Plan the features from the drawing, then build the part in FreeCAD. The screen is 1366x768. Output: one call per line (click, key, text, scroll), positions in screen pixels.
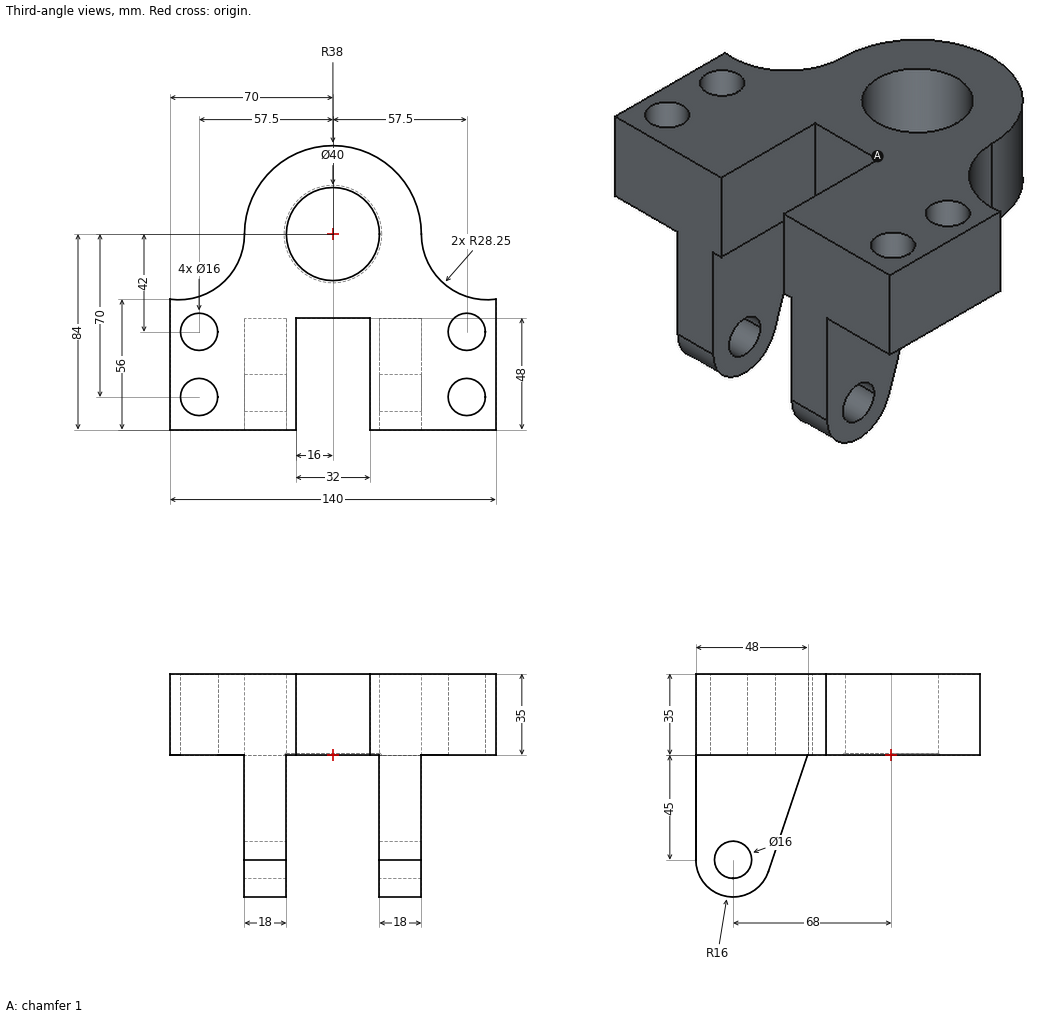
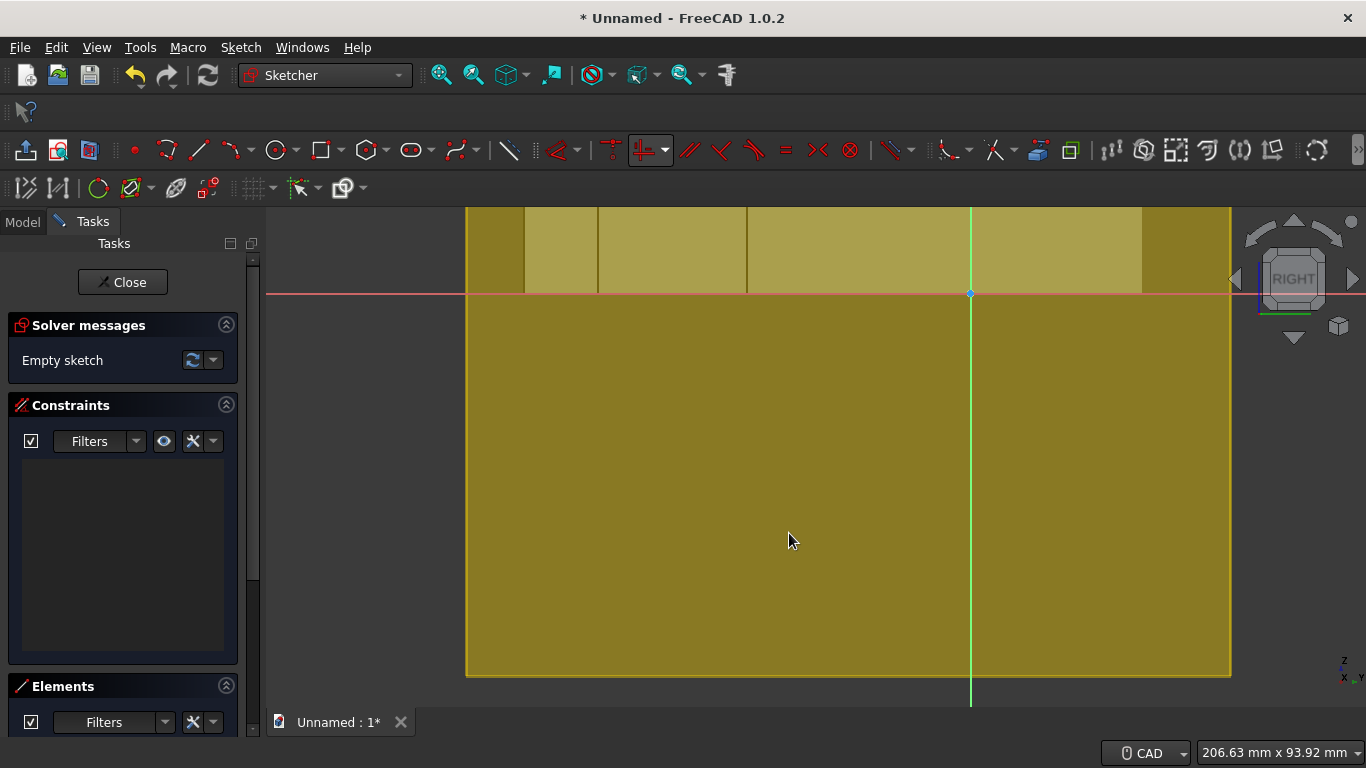
click(168, 150)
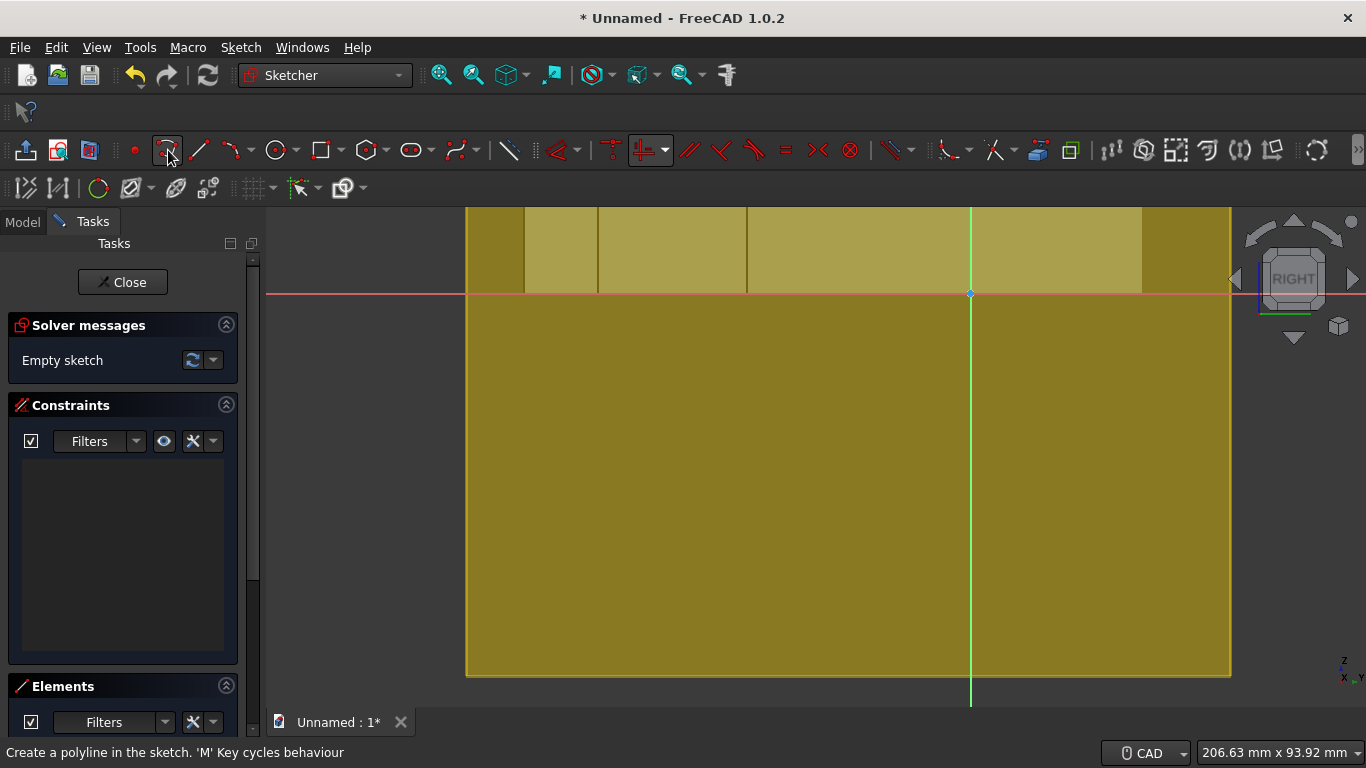
click(690, 561)
click(779, 294)
click(524, 303)
click(524, 534)
right_click(524, 534)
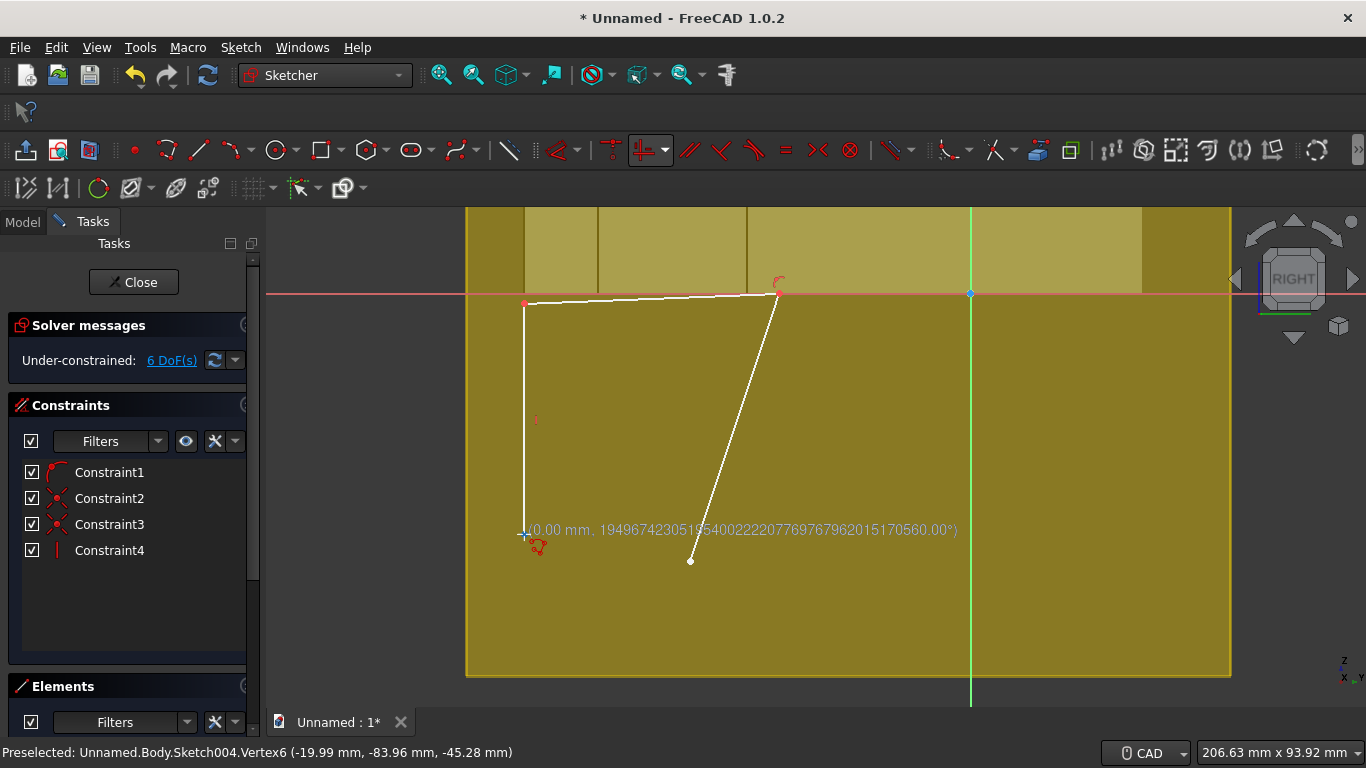
click(232, 150)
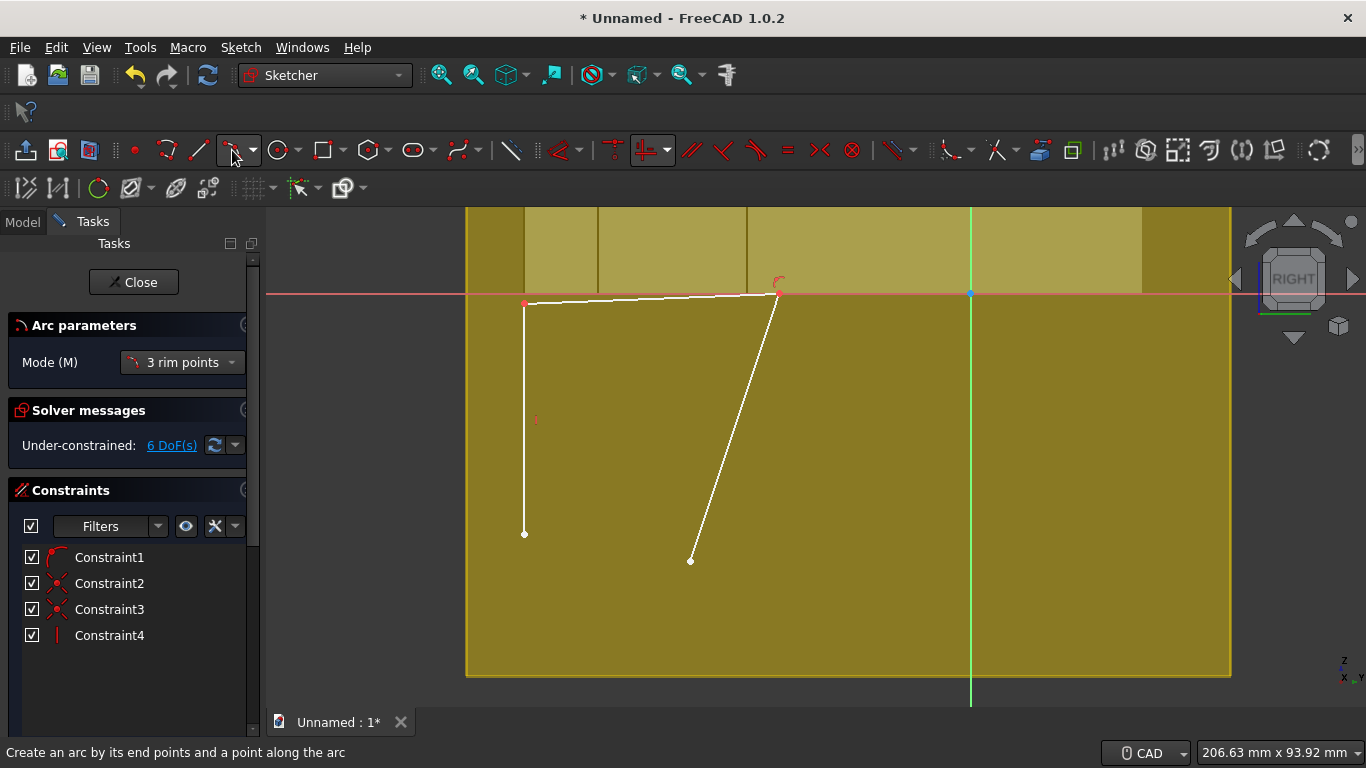
click(524, 535)
click(690, 562)
click(595, 618)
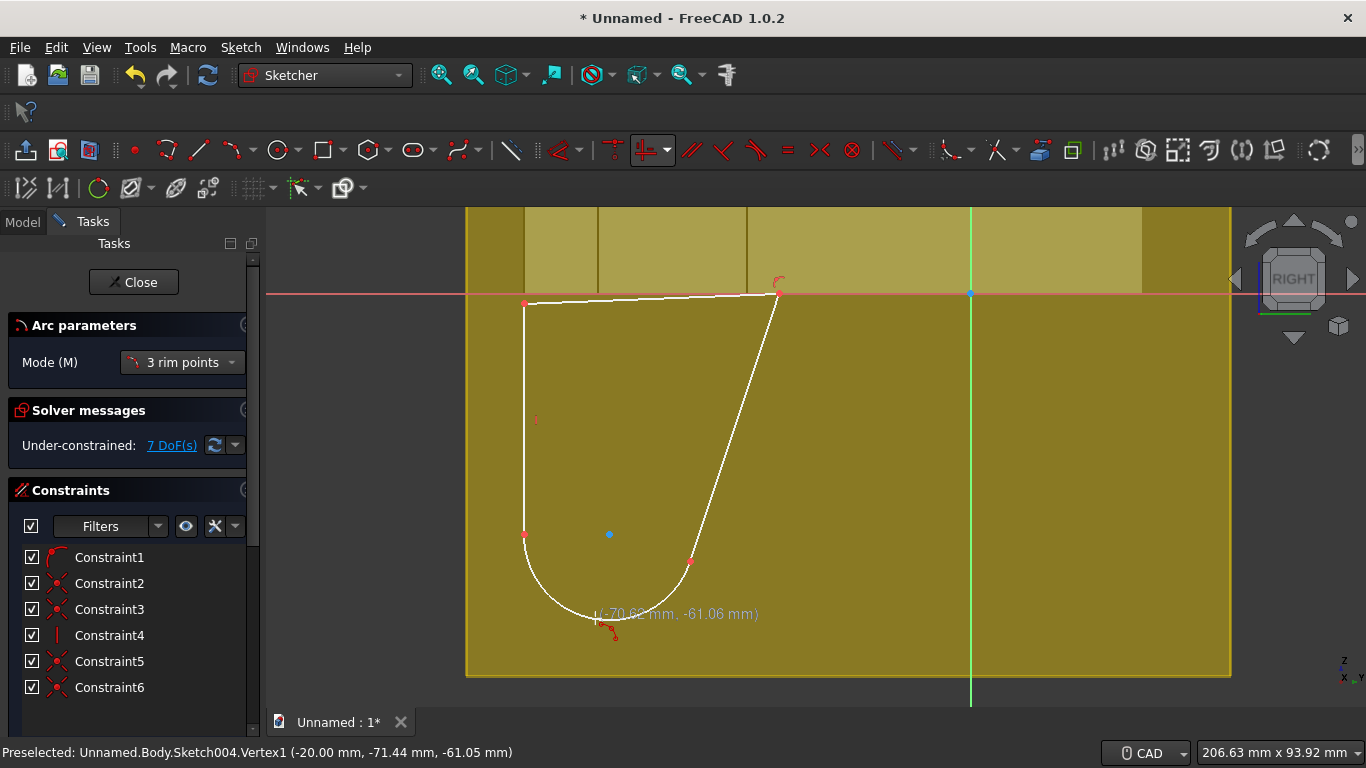
key(g)
key(c)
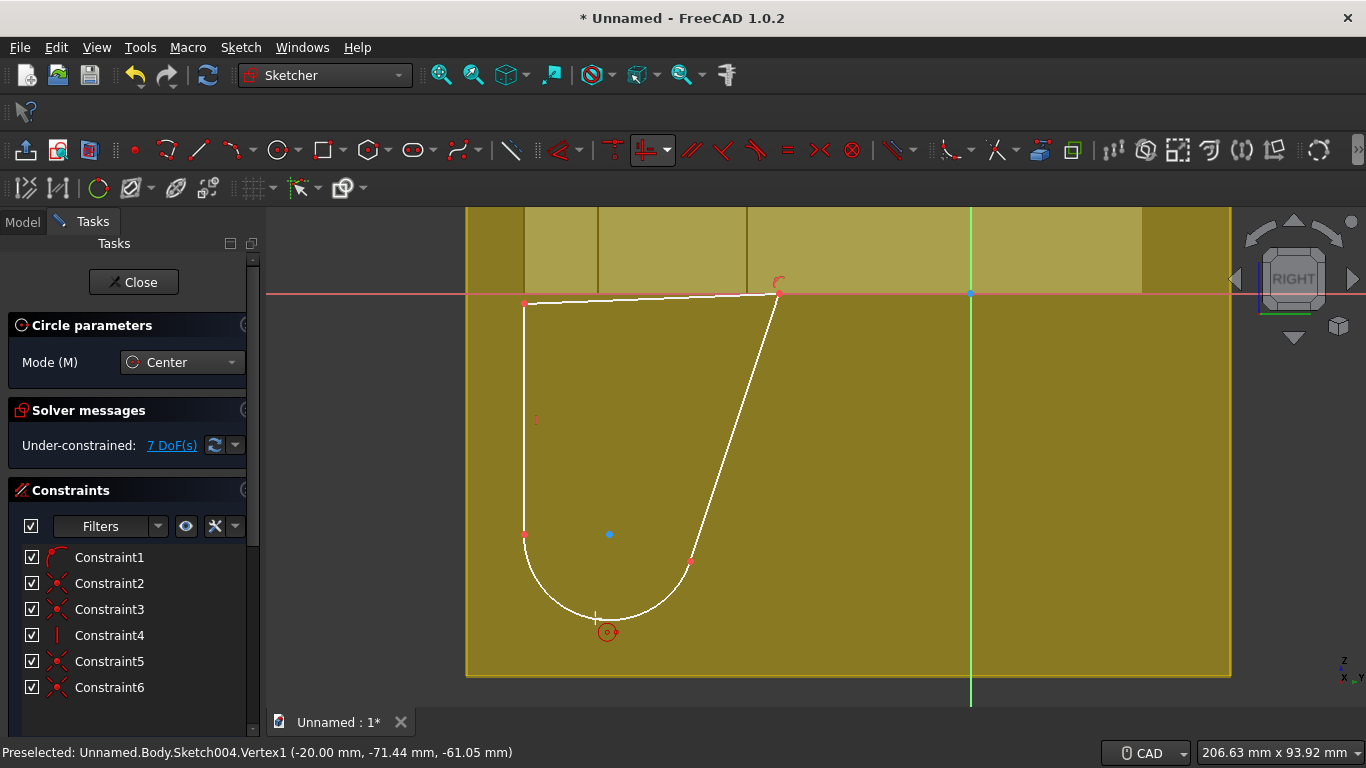
click(609, 534)
move(639, 503)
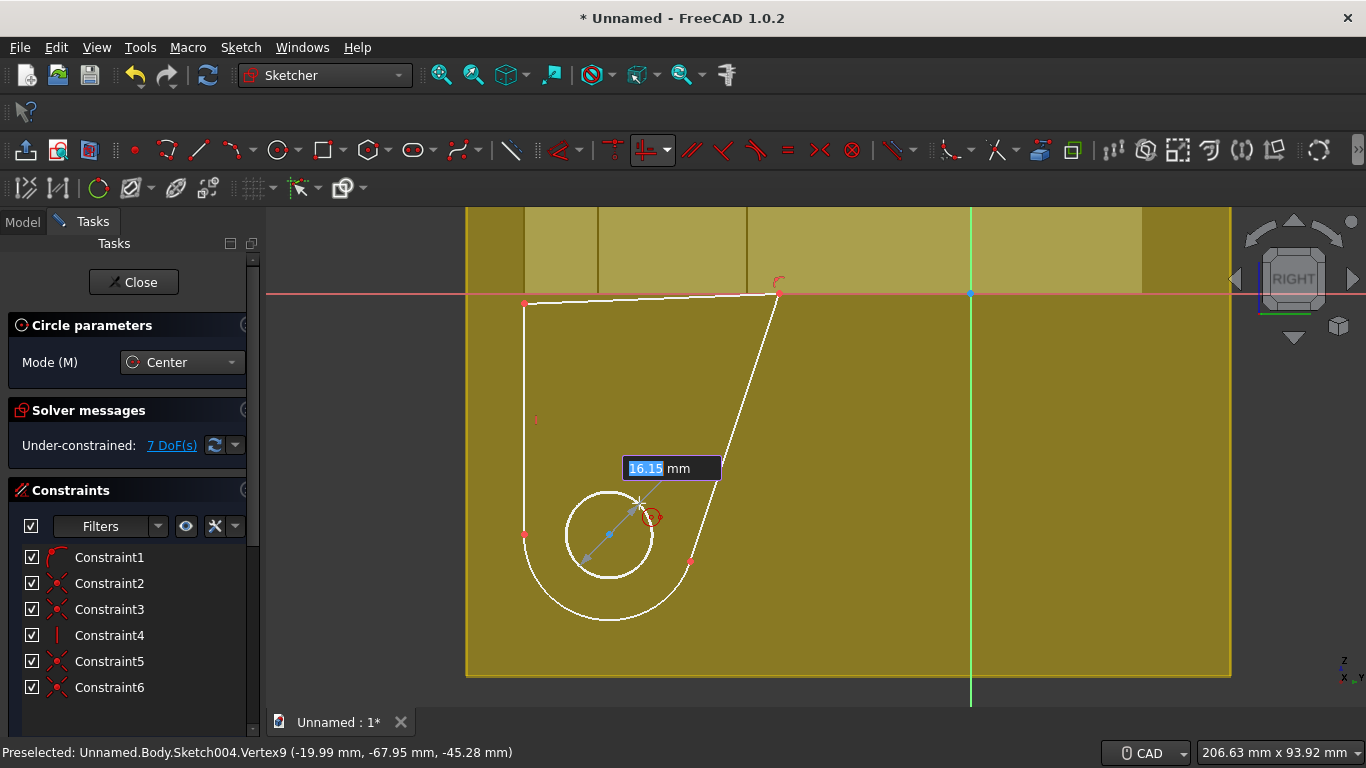
text(16)
key(Return)
key(Escape)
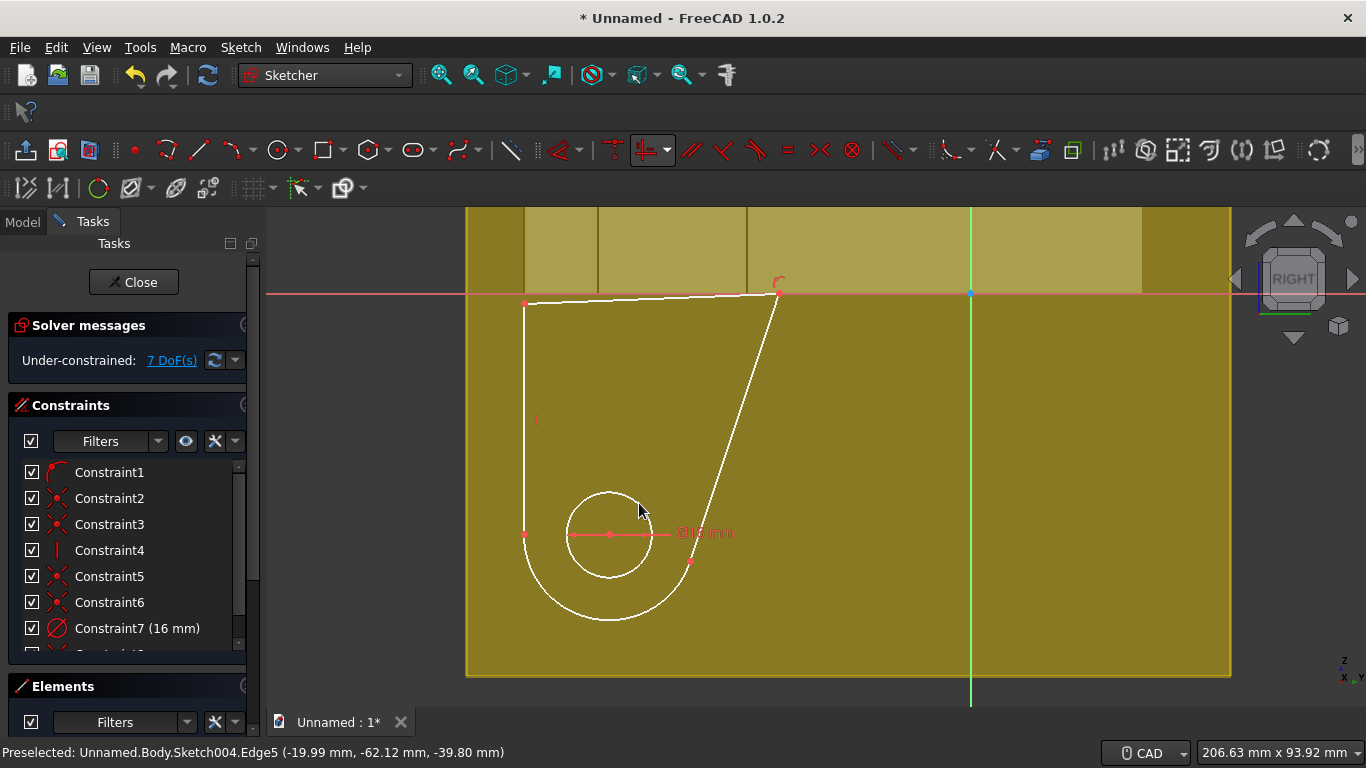
click(717, 482)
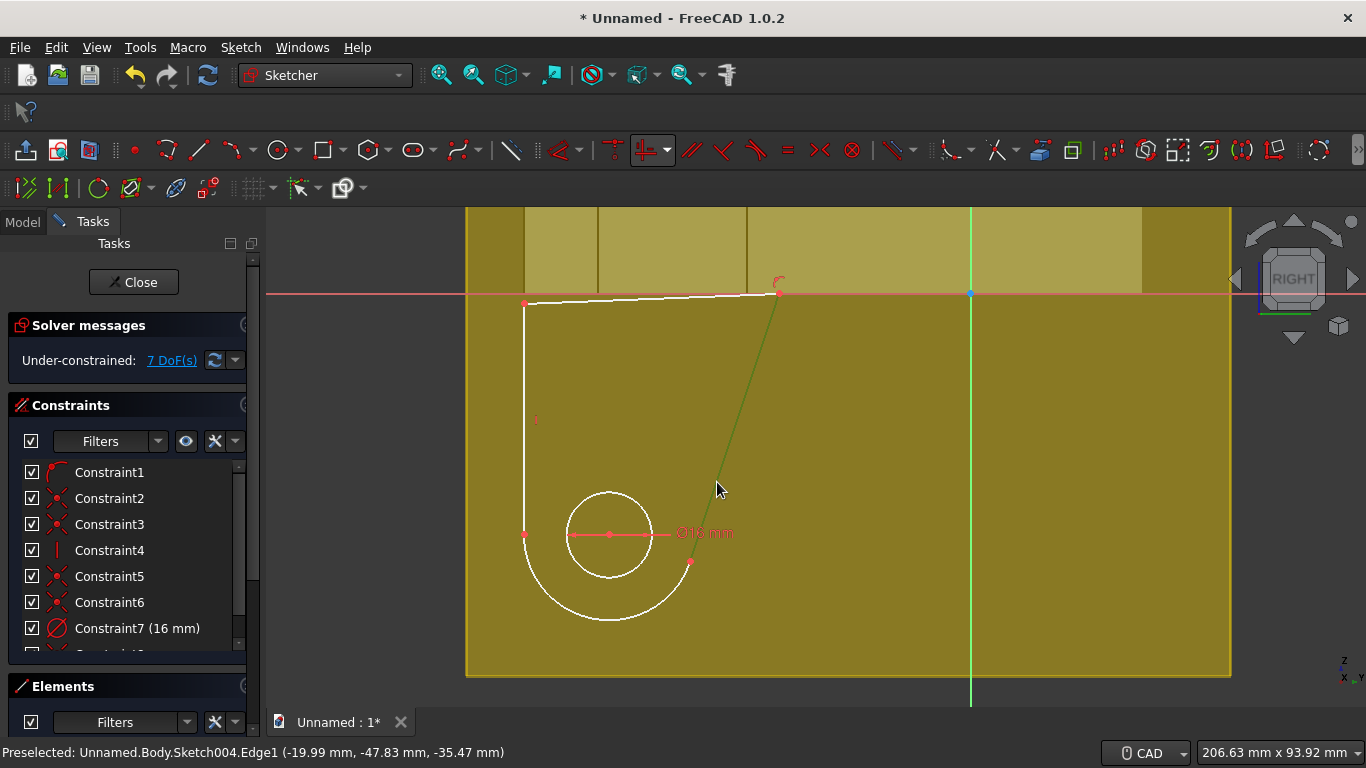
click(553, 599)